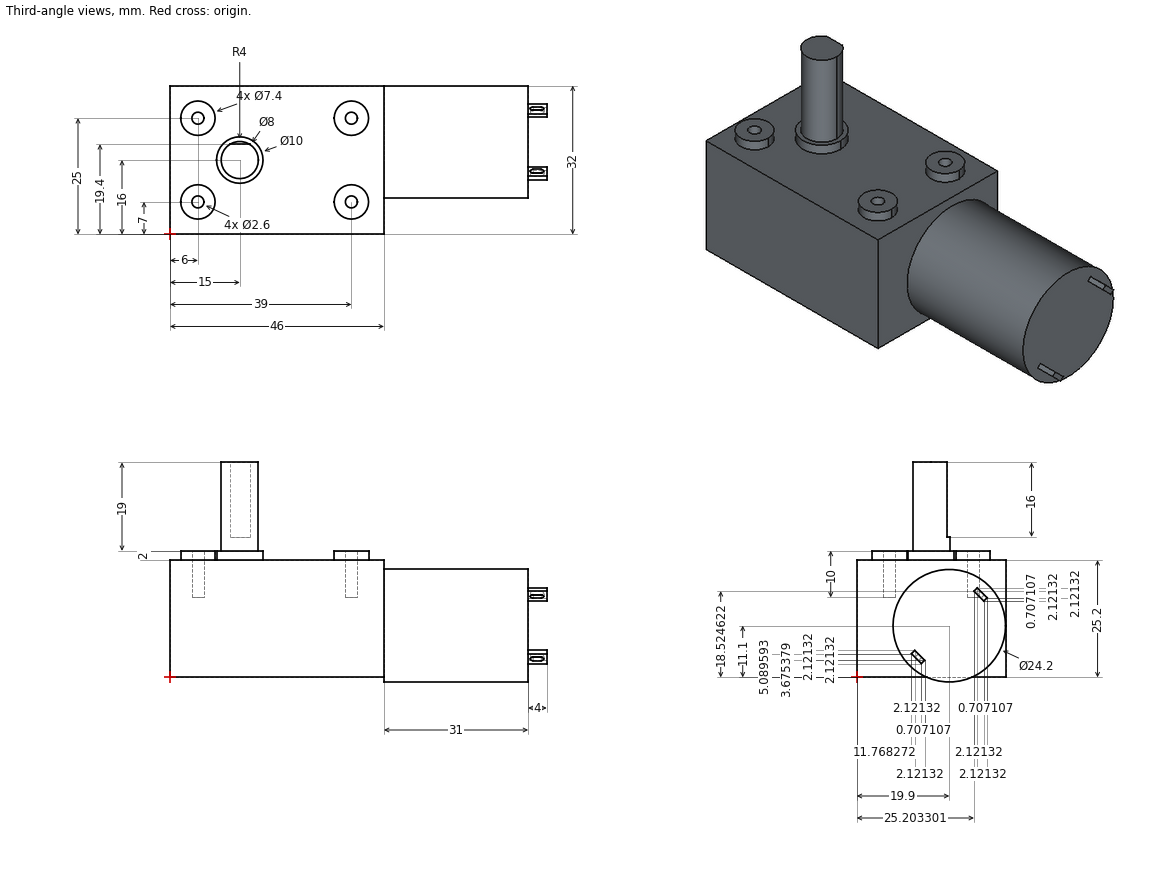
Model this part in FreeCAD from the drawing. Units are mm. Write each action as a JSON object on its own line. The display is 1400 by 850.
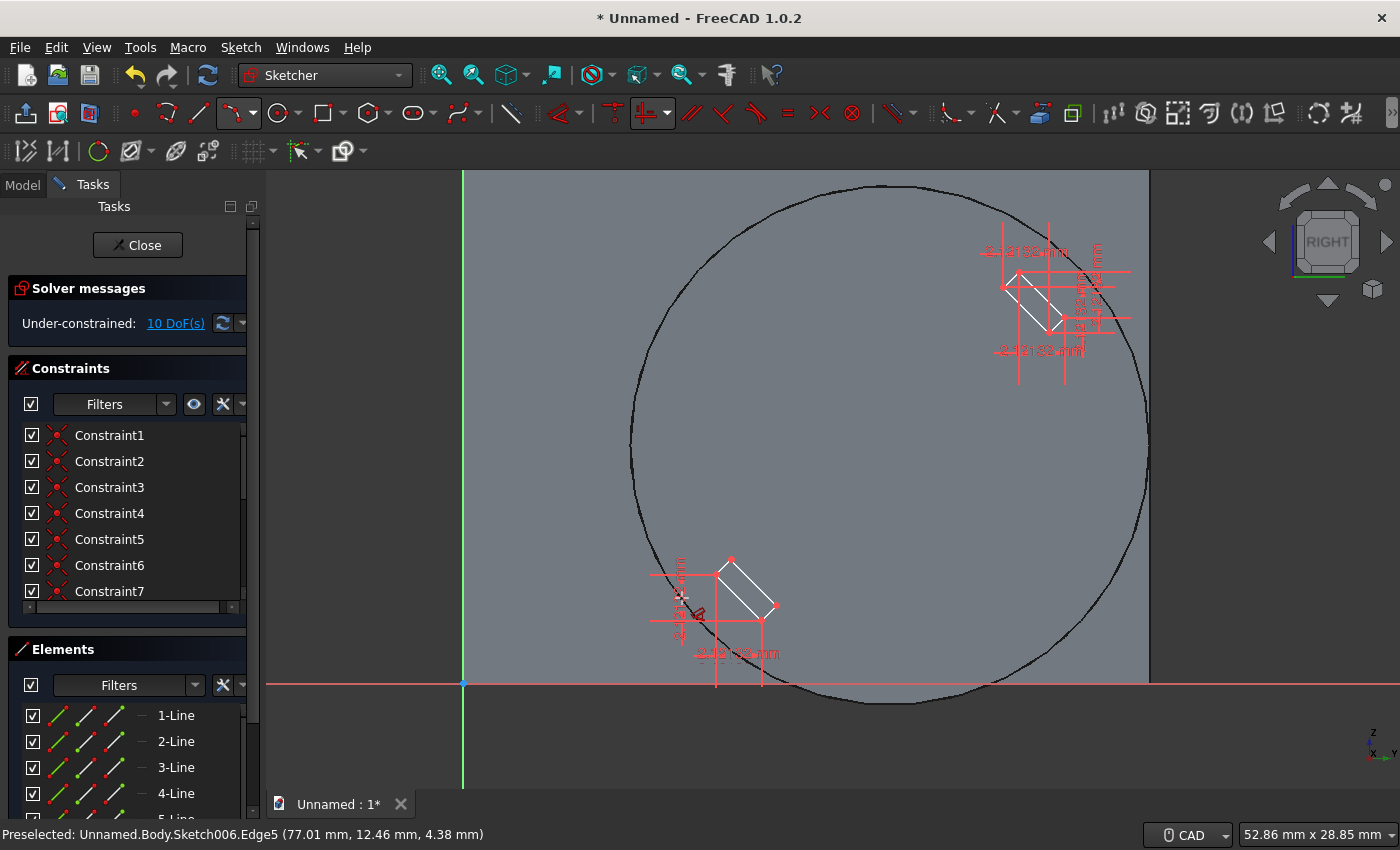
{"action": "left_click", "coordinate": [763, 592]}
{"action": "left_click", "coordinate": [753, 526]}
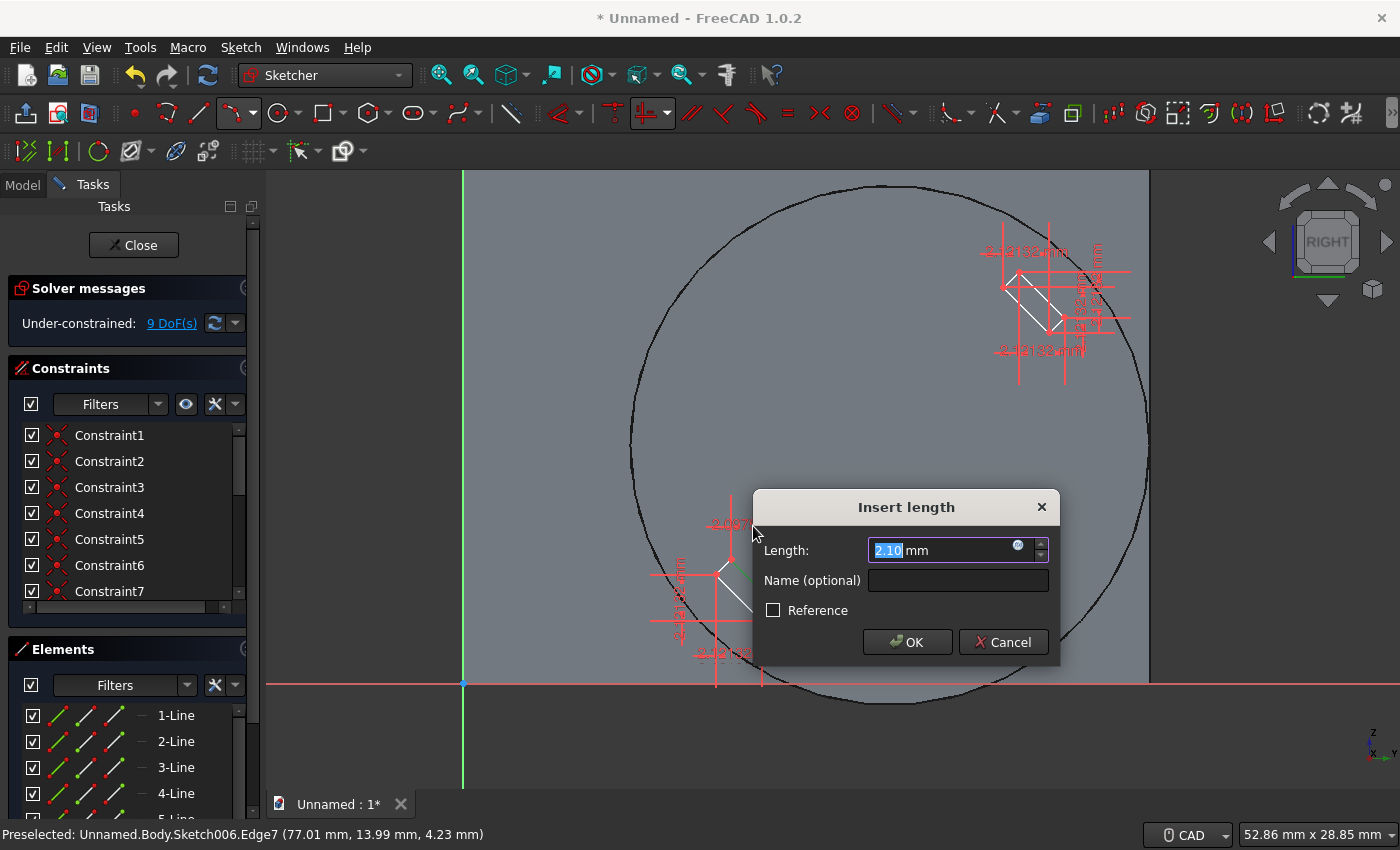
{"action": "type", "text": "2.12132"}
{"action": "key", "text": "Return"}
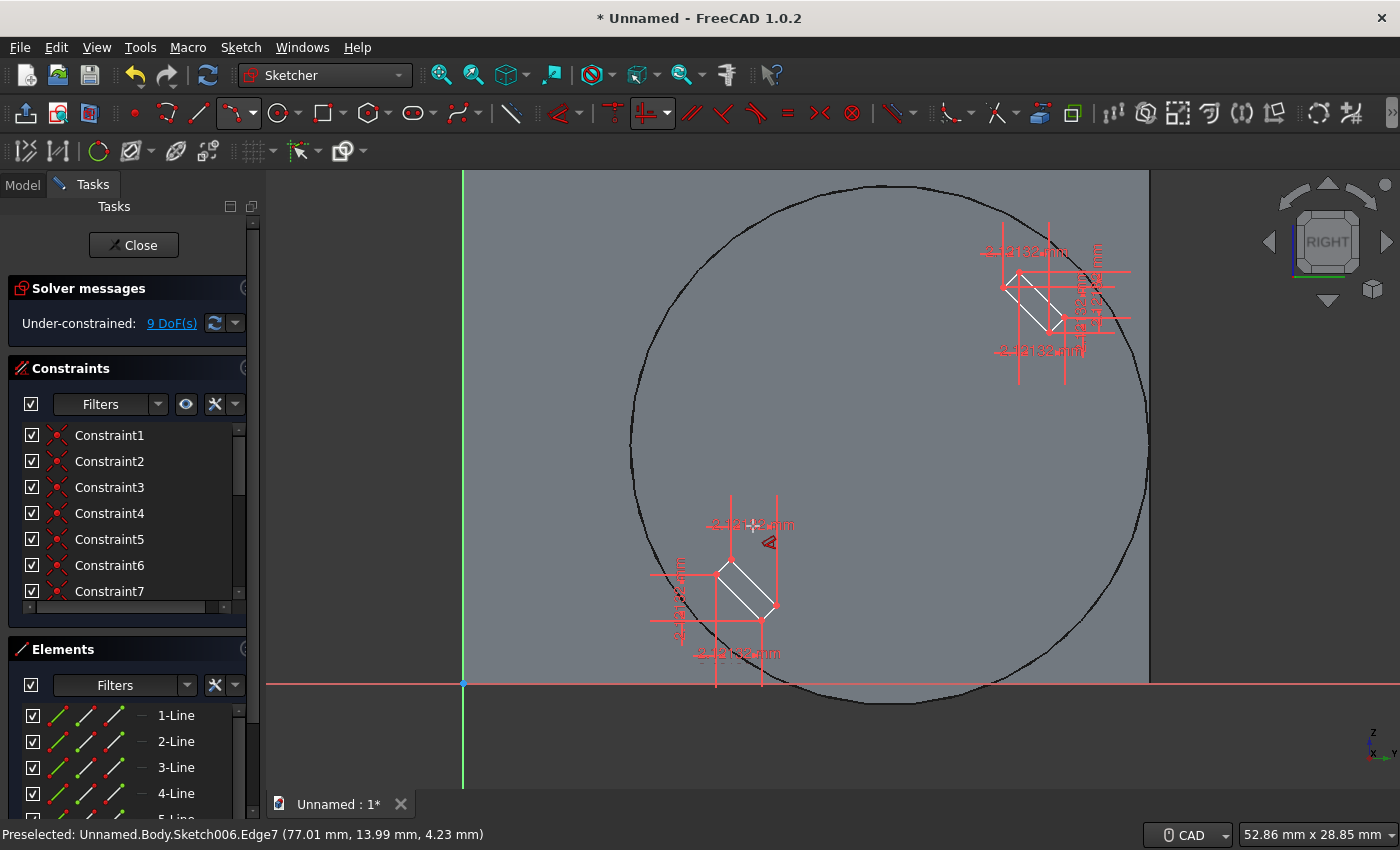
{"action": "left_click", "coordinate": [763, 592]}
{"action": "left_click", "coordinate": [697, 572]}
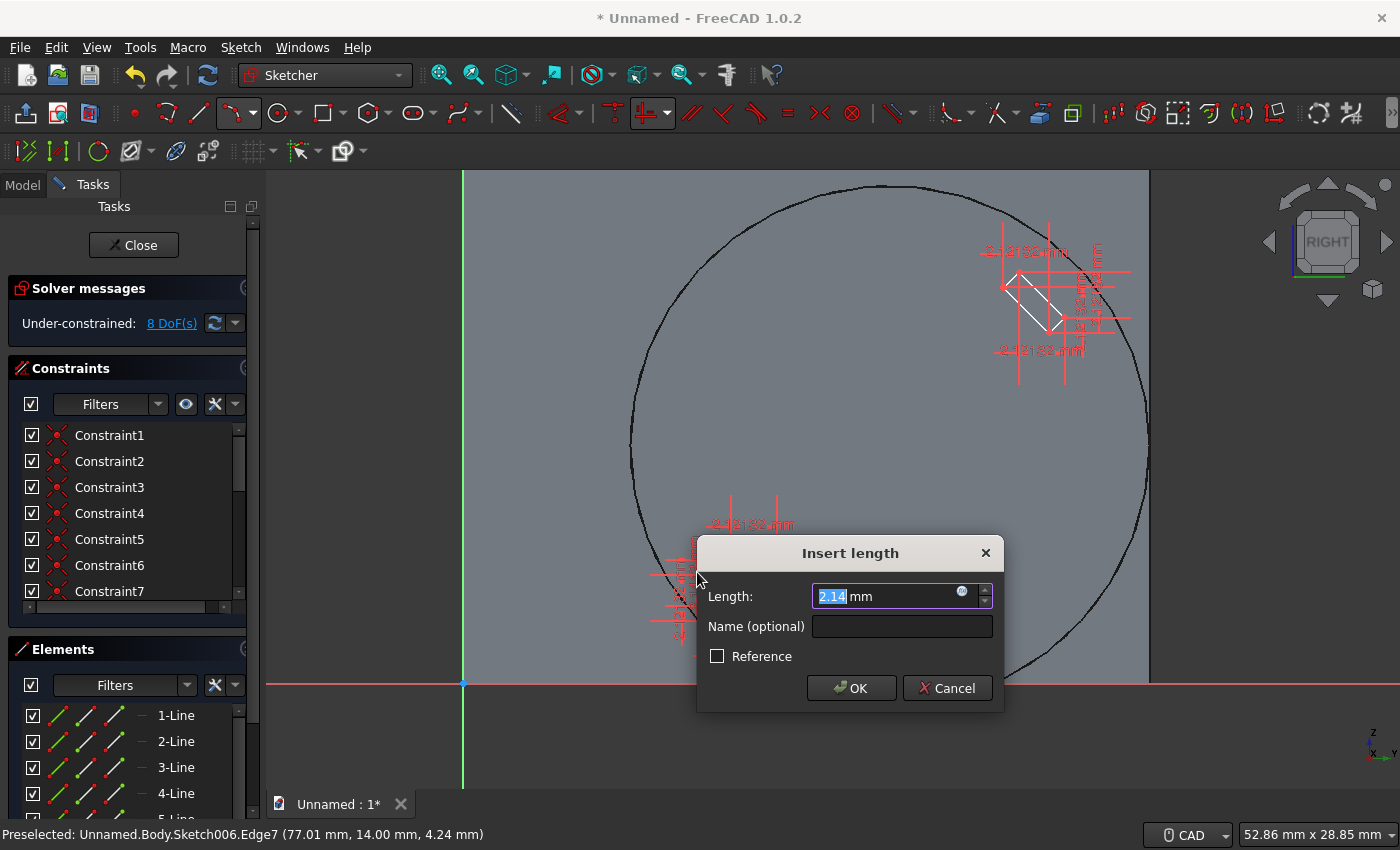
{"action": "type", "text": "2.12132"}
{"action": "key", "text": "Return"}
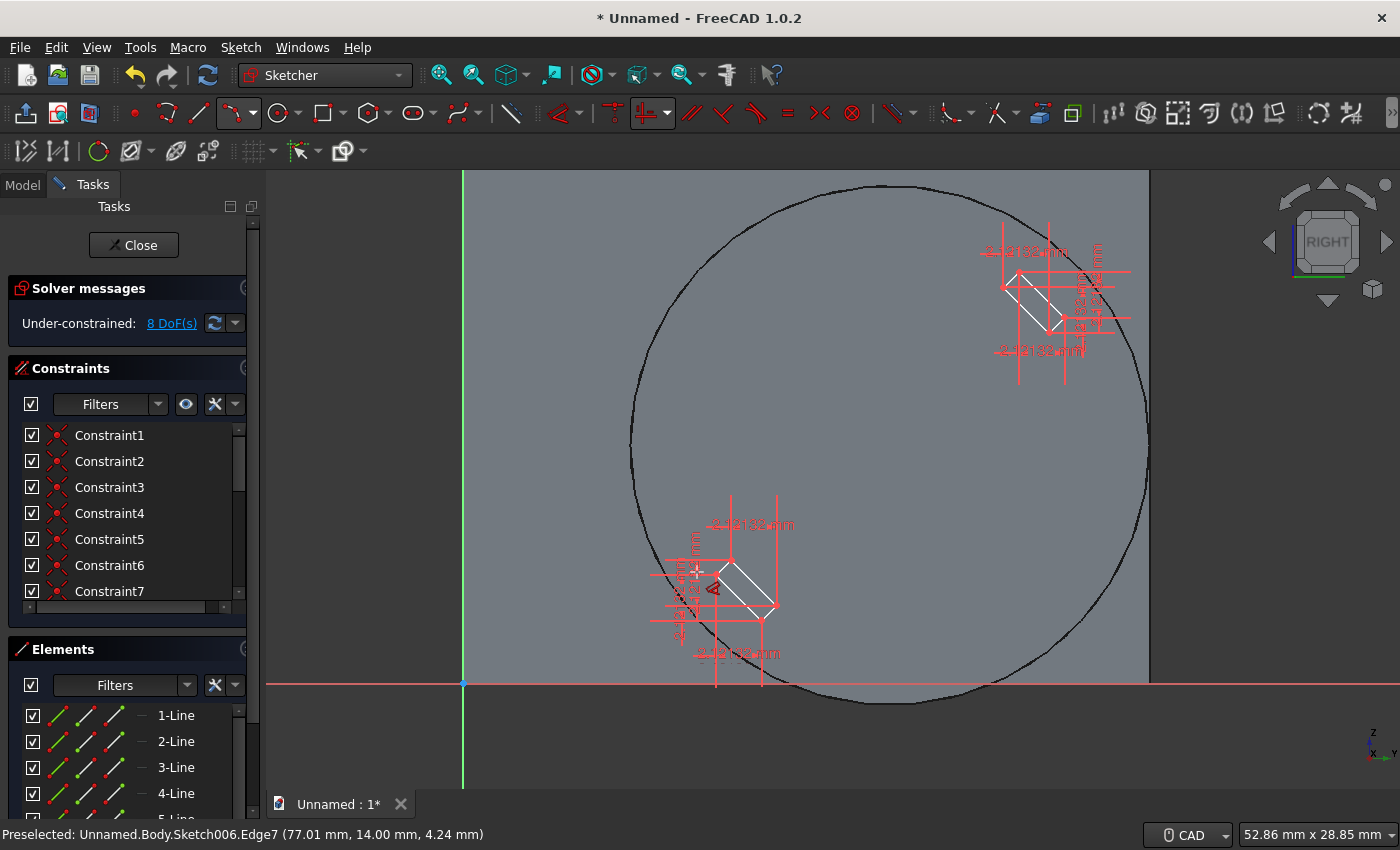
{"action": "left_click", "coordinate": [716, 575]}
{"action": "left_click", "coordinate": [429, 629]}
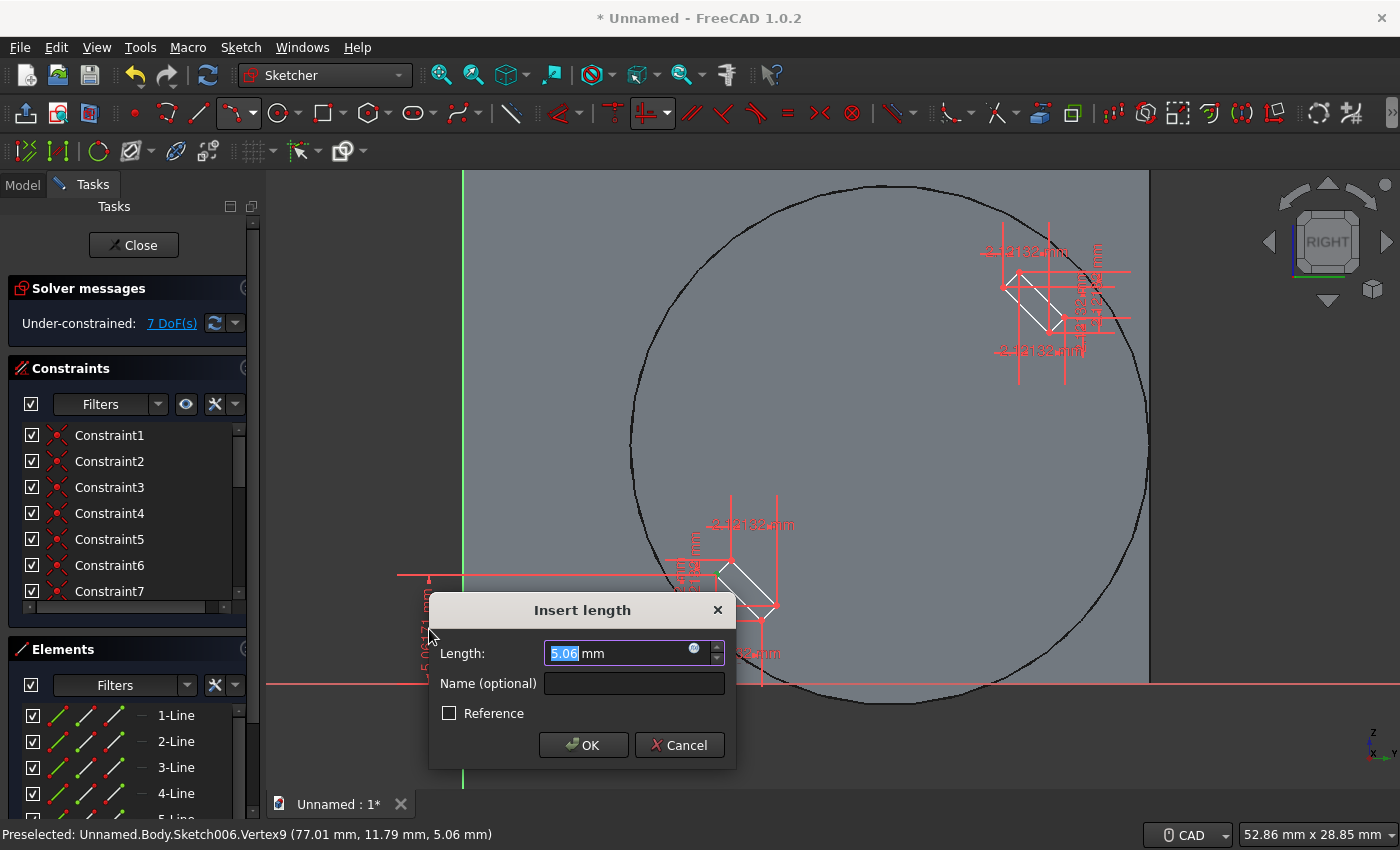
{"action": "type", "text": "5.089593"}
{"action": "key", "text": "Return"}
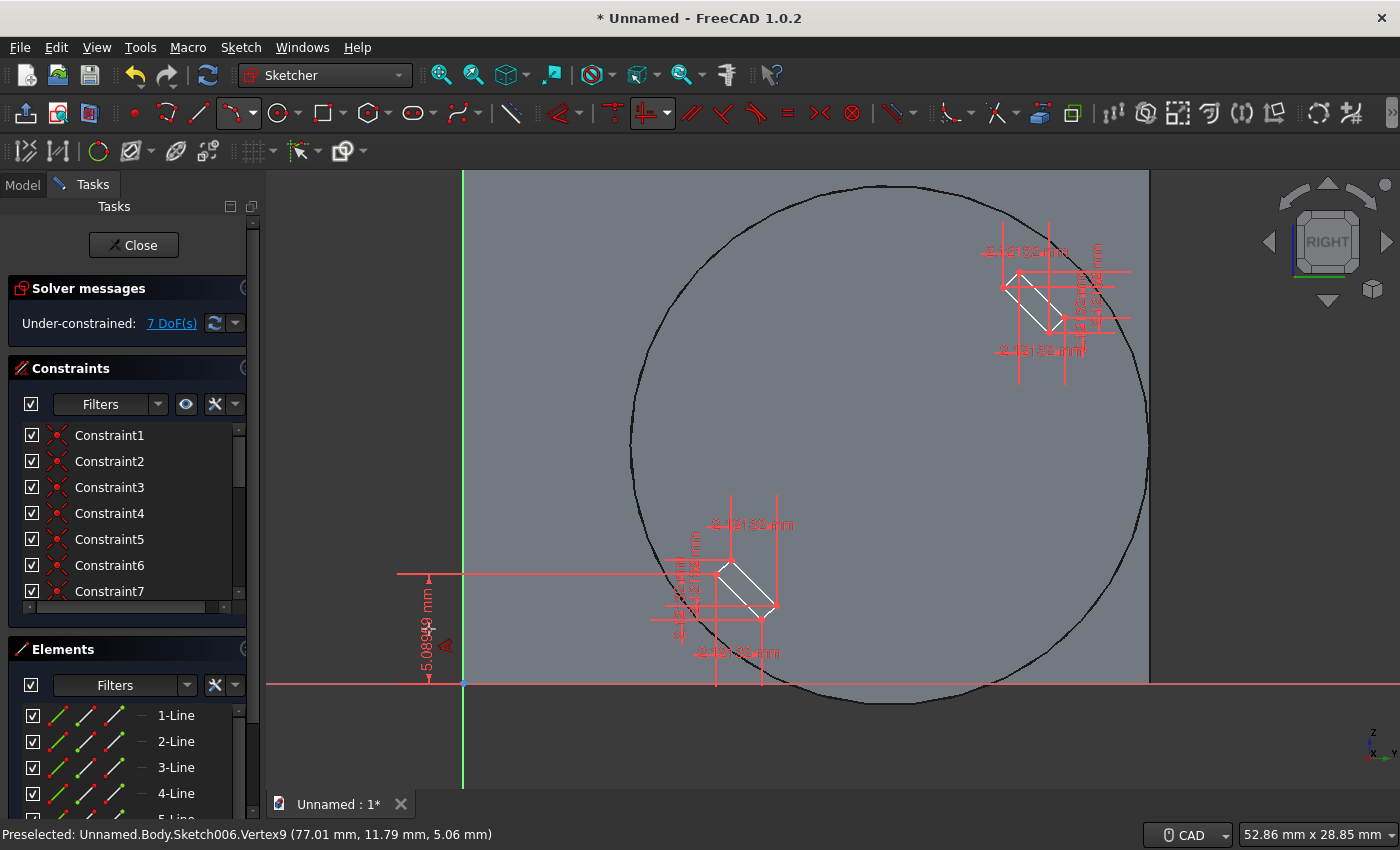
{"action": "left_click", "coordinate": [777, 606]}
{"action": "left_click", "coordinate": [429, 663]}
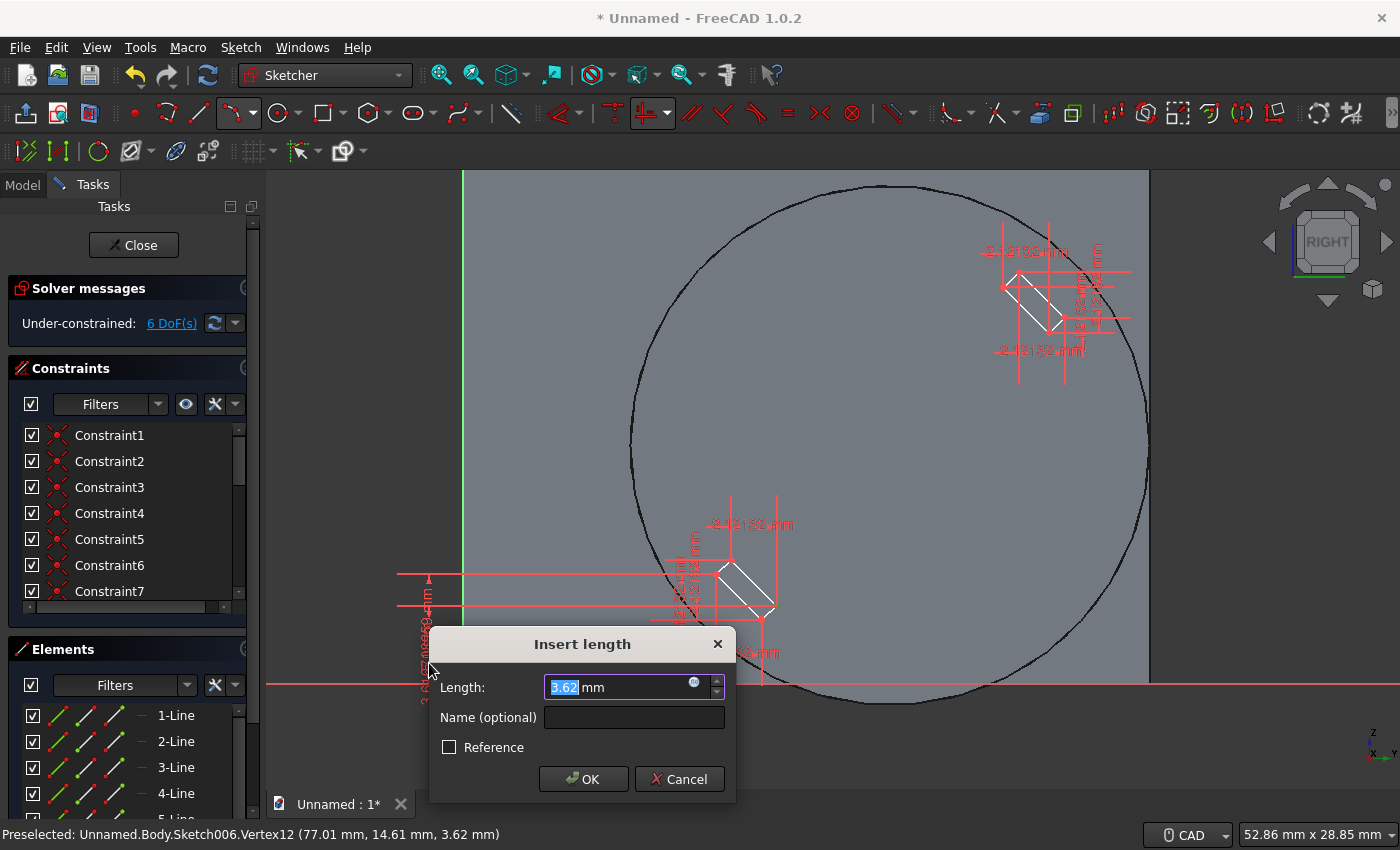
{"action": "type", "text": "3.675379"}
{"action": "key", "text": "Return"}